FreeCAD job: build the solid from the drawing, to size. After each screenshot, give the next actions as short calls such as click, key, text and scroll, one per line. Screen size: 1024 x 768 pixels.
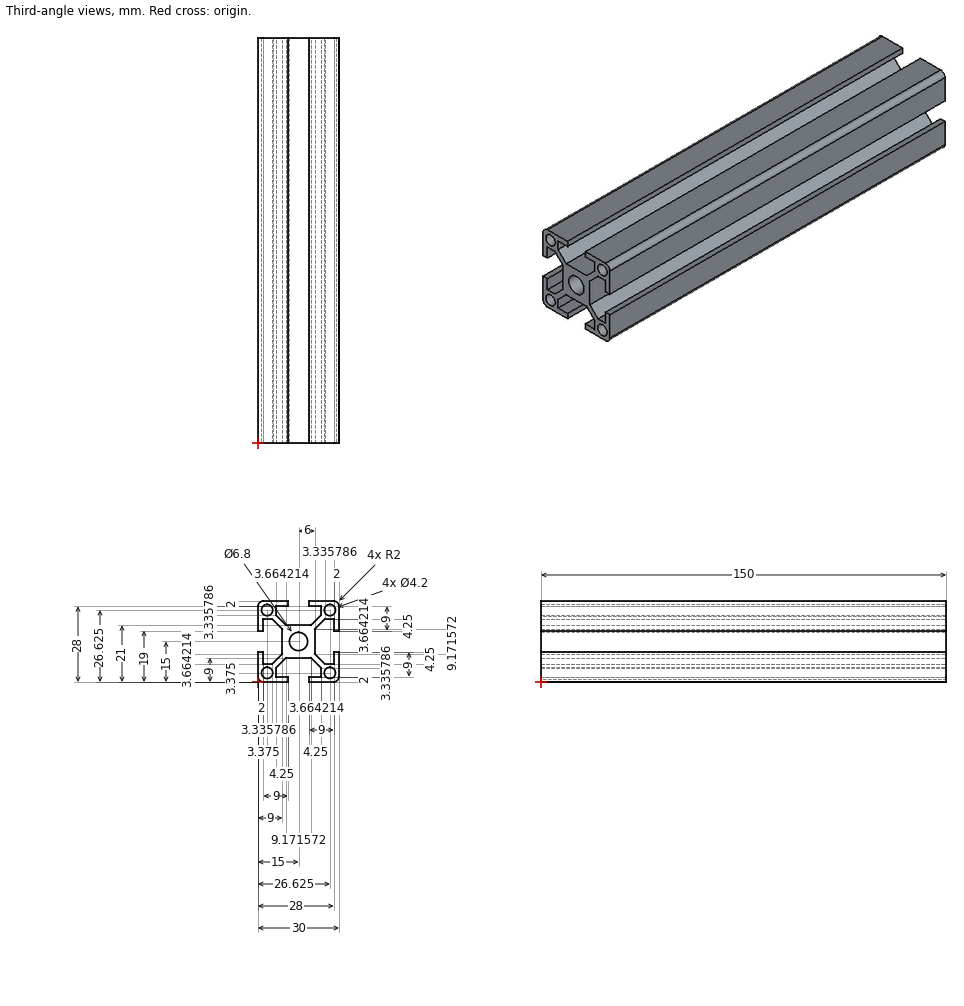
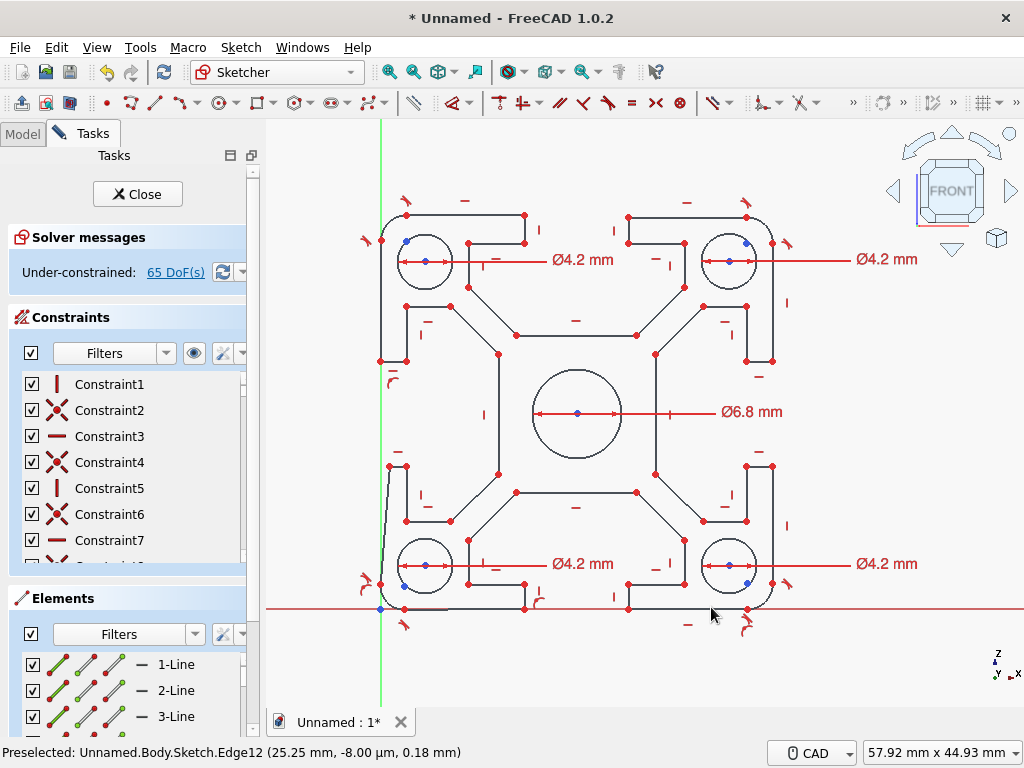
click(489, 609)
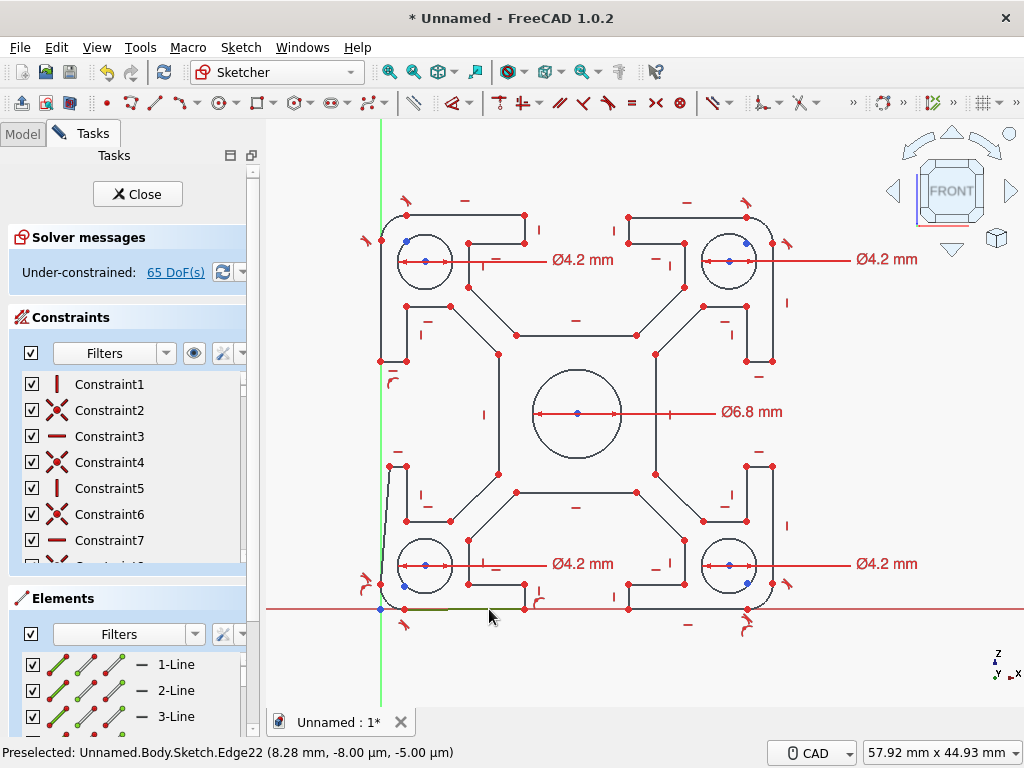
click(542, 104)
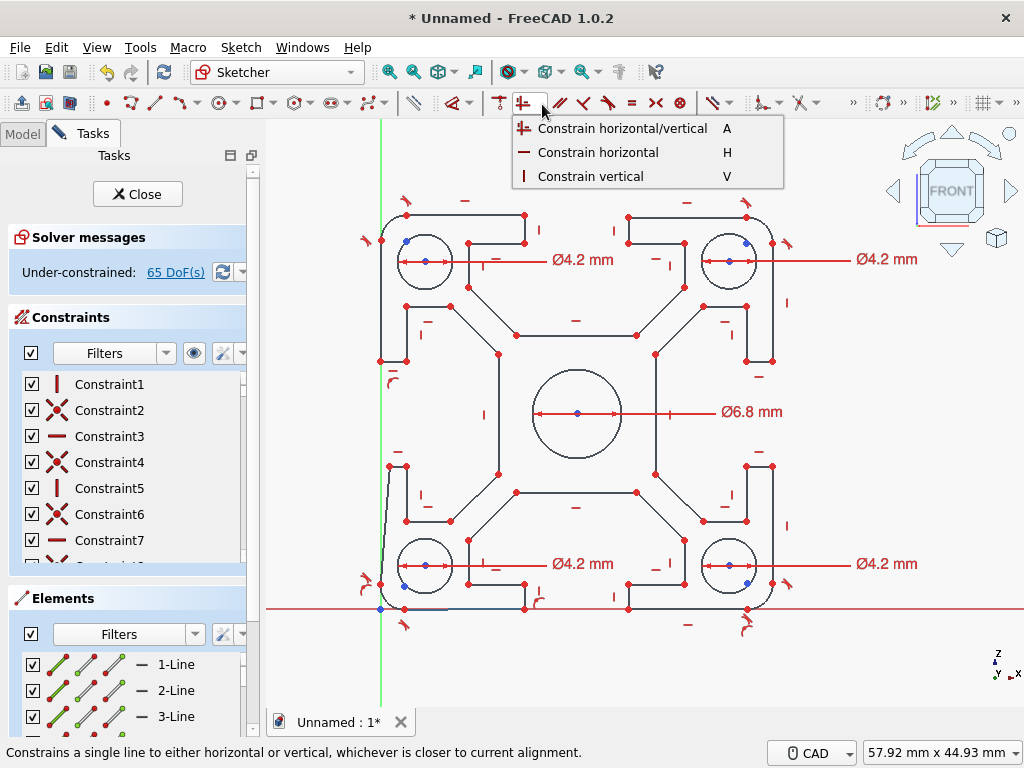
click(648, 152)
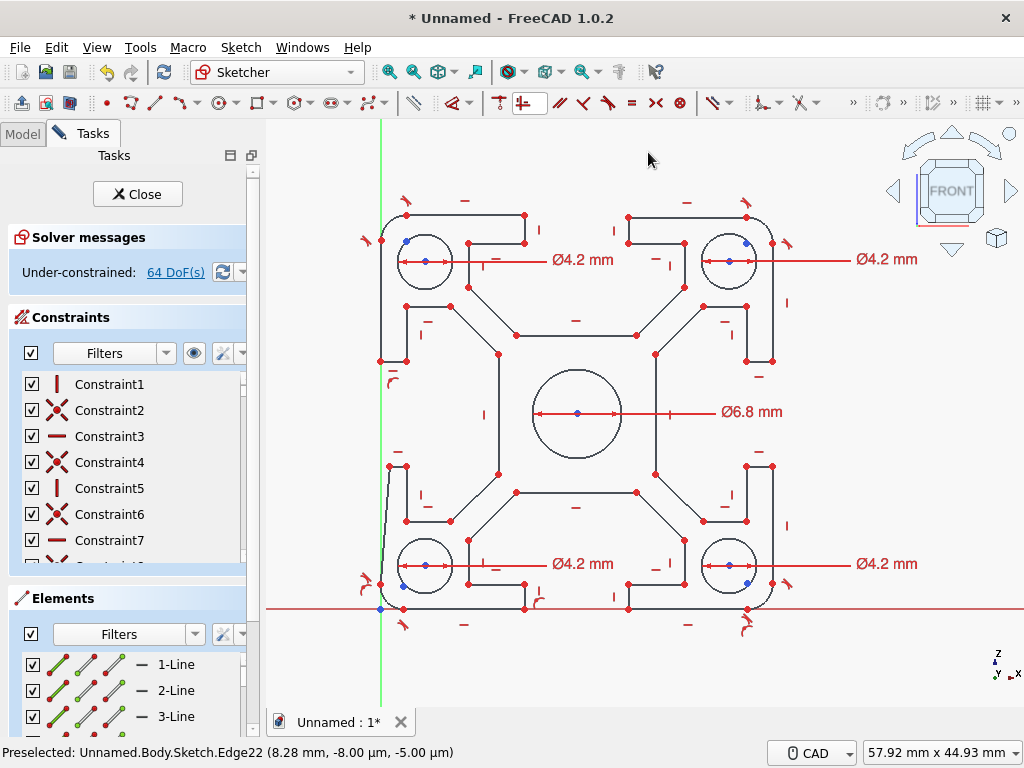
click(383, 549)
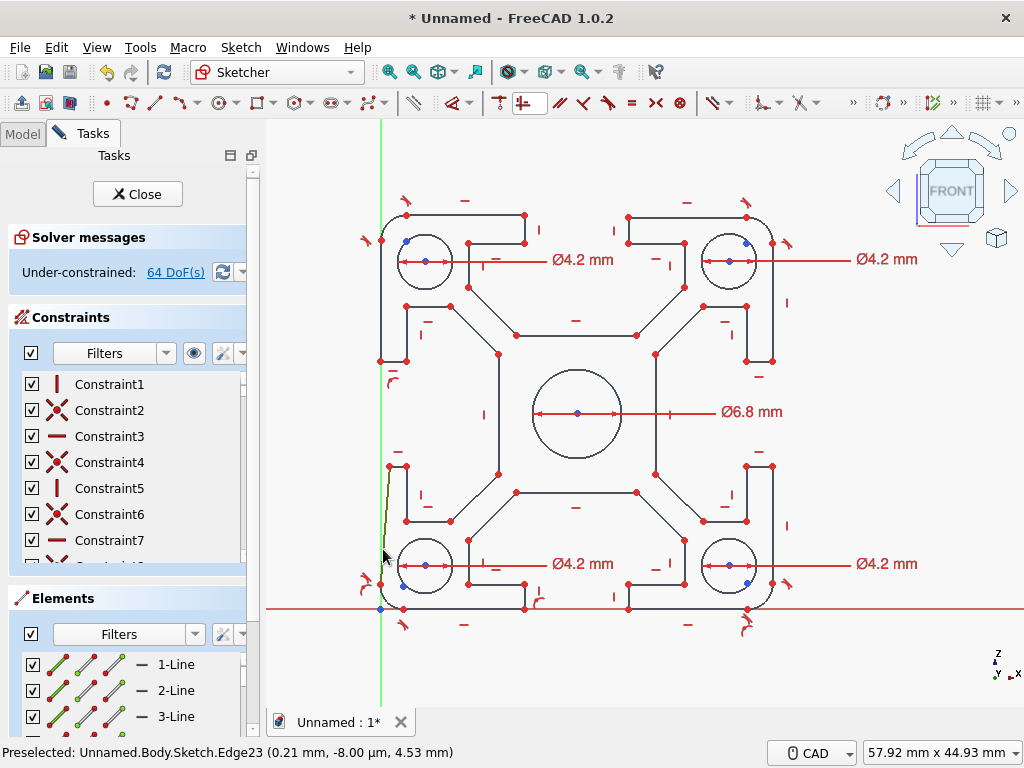
key(v)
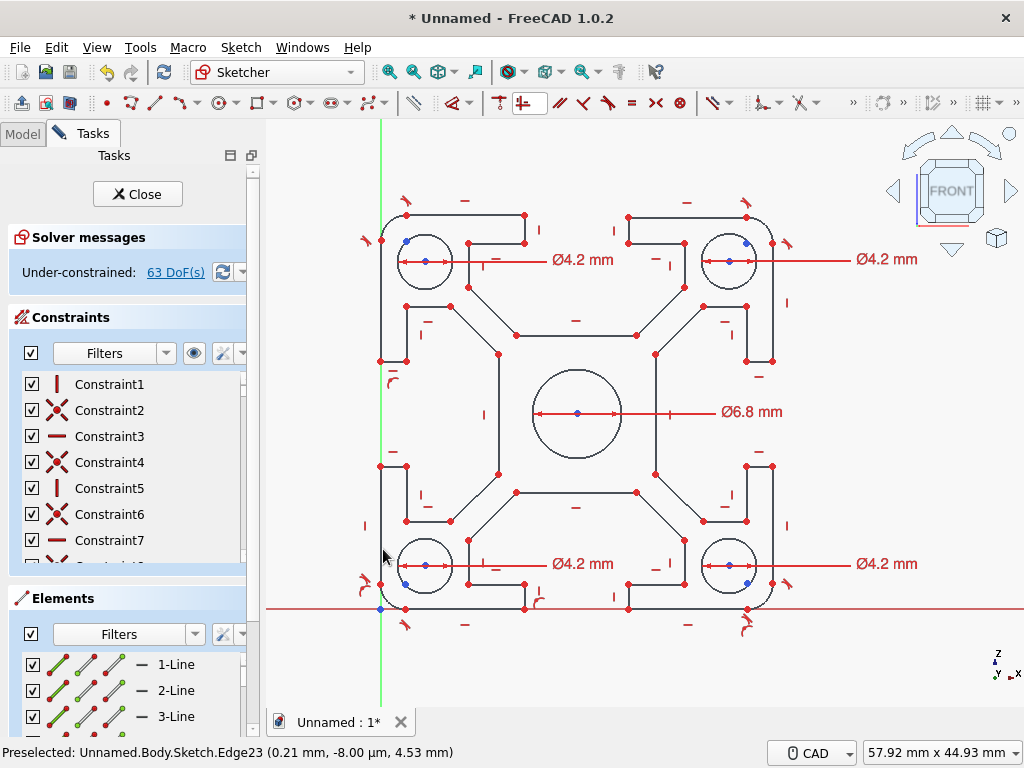
click(381, 325)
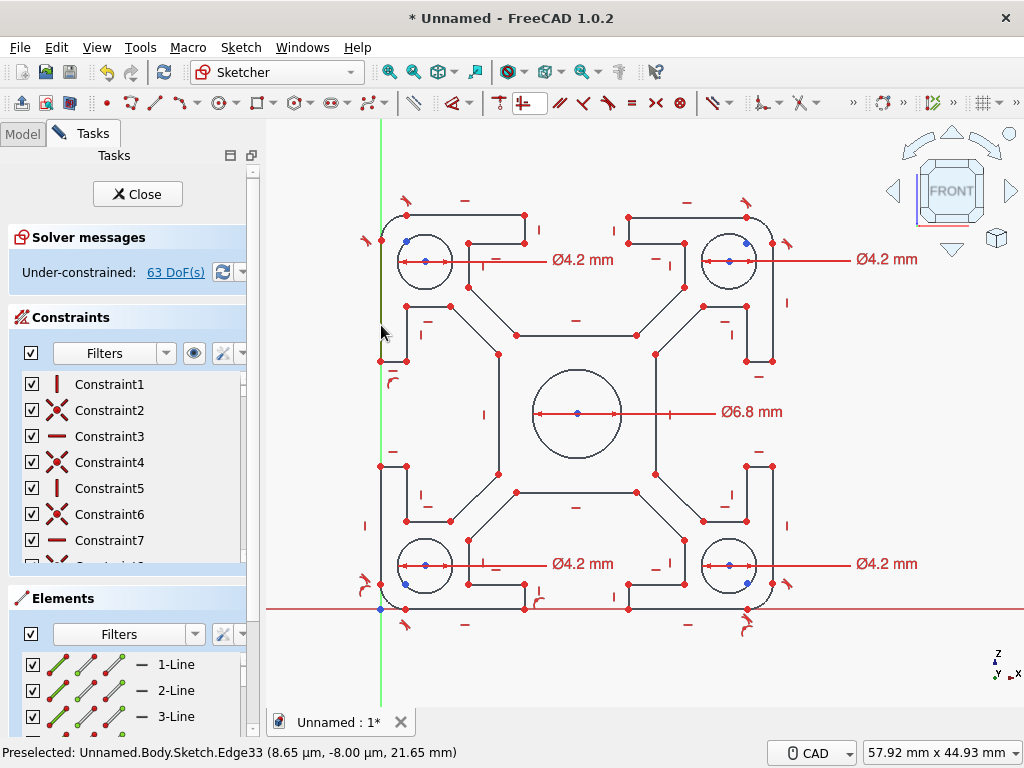
click(542, 104)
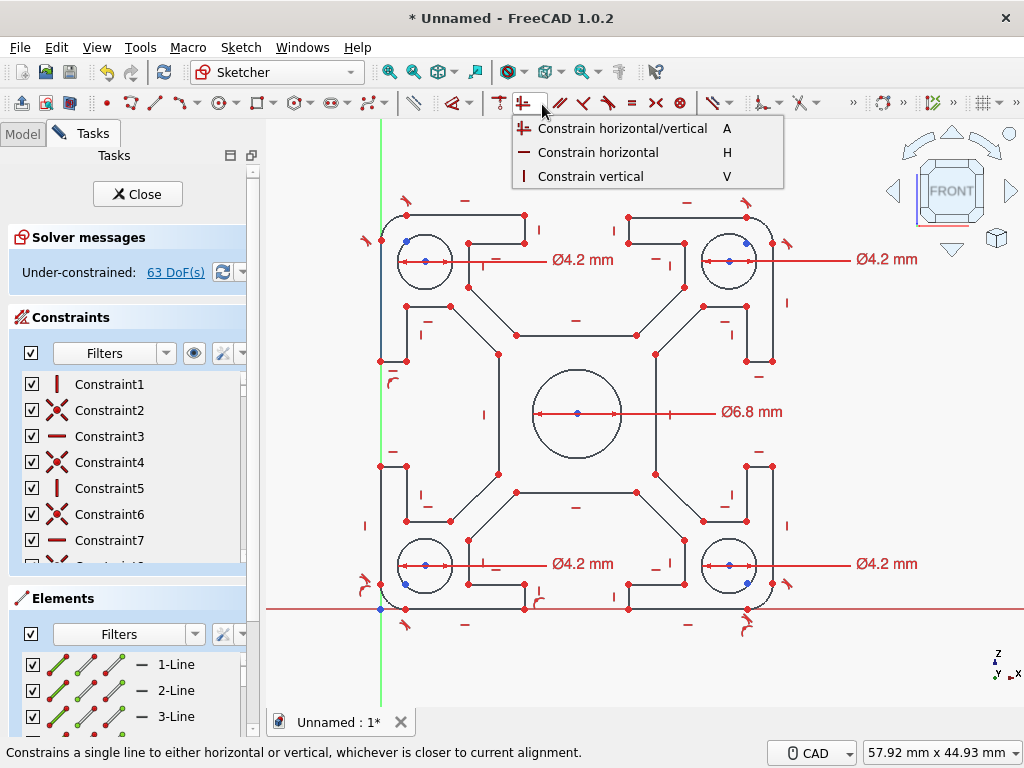
click(648, 176)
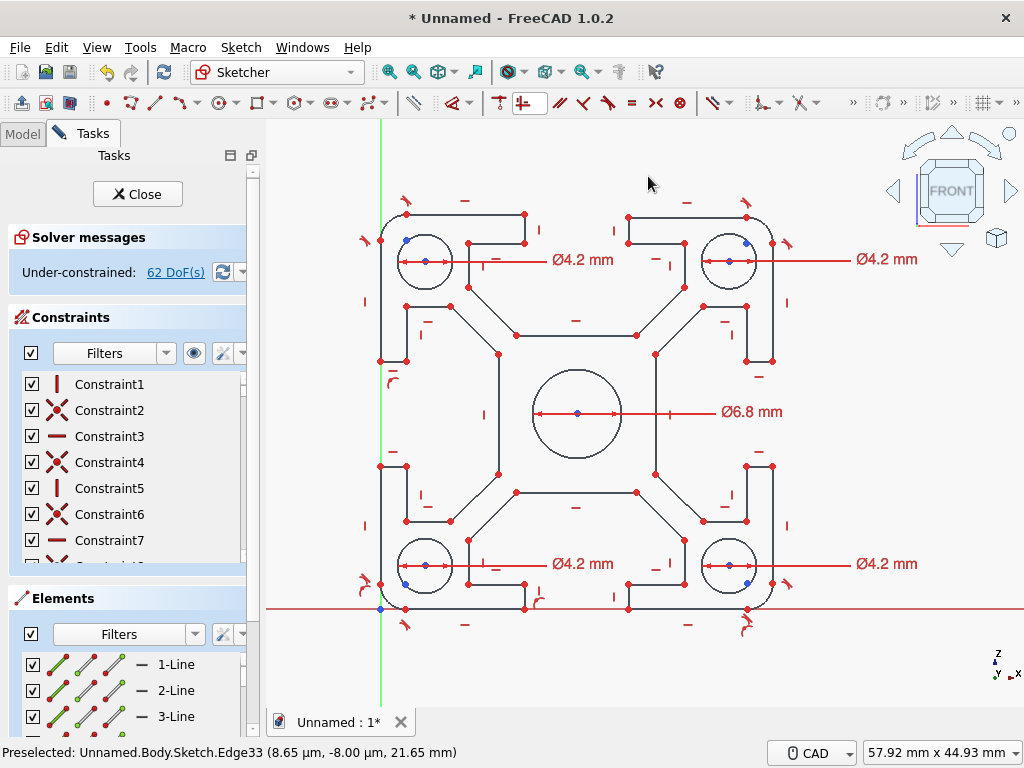
click(759, 607)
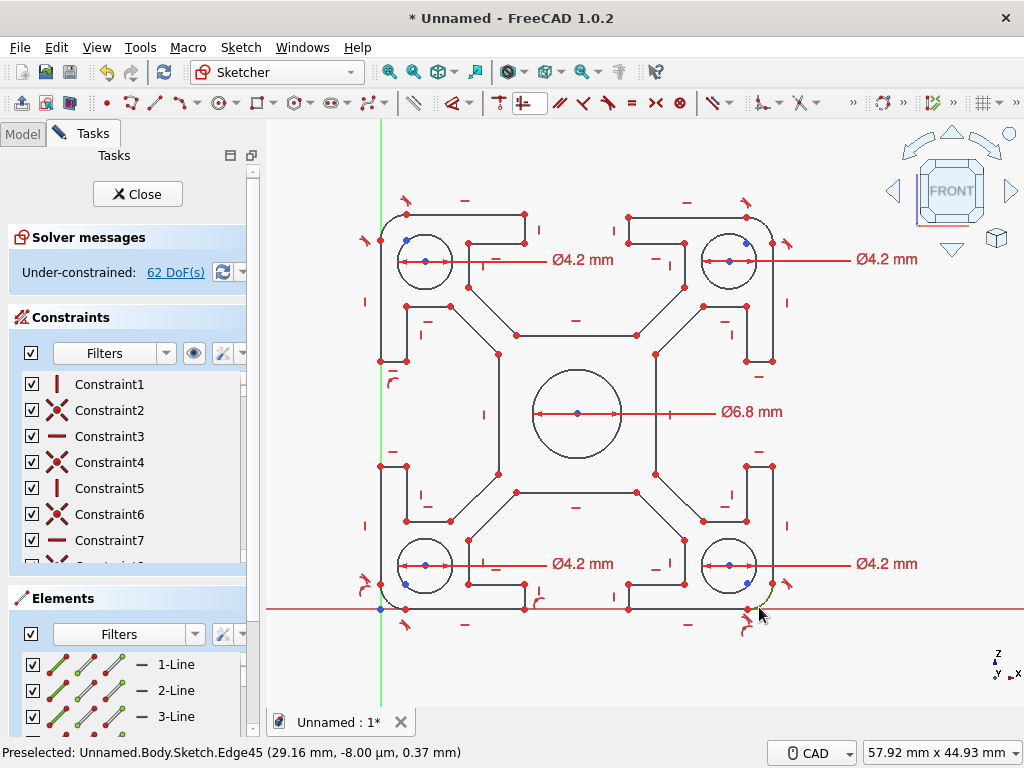
click(383, 596)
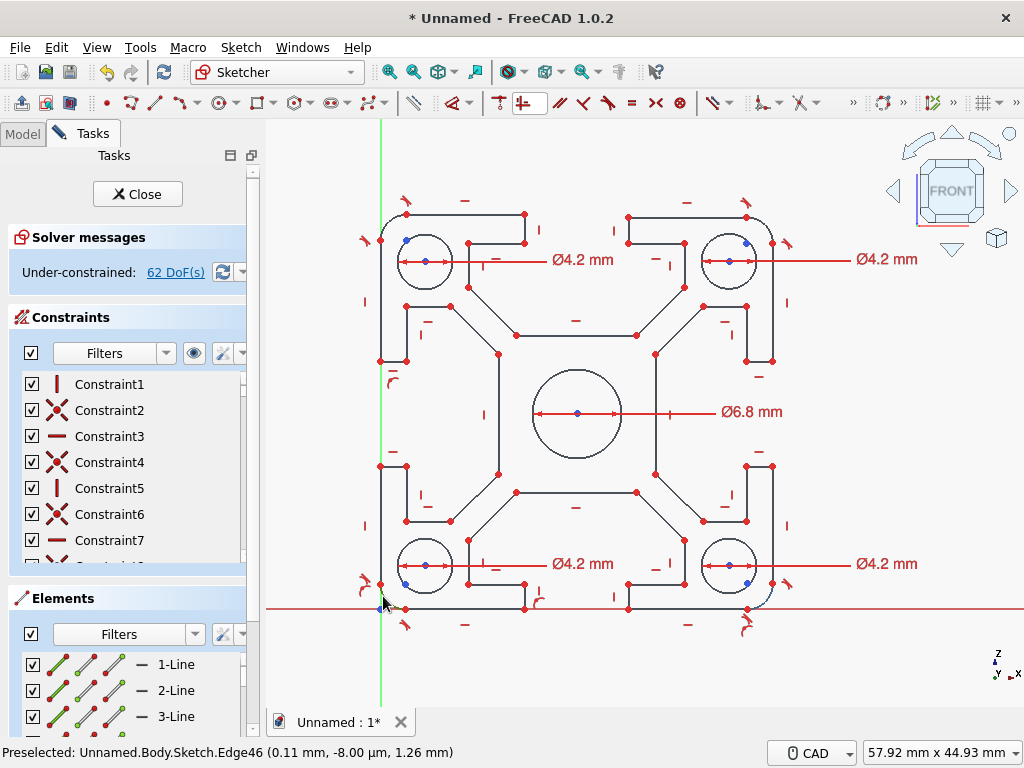
click(395, 218)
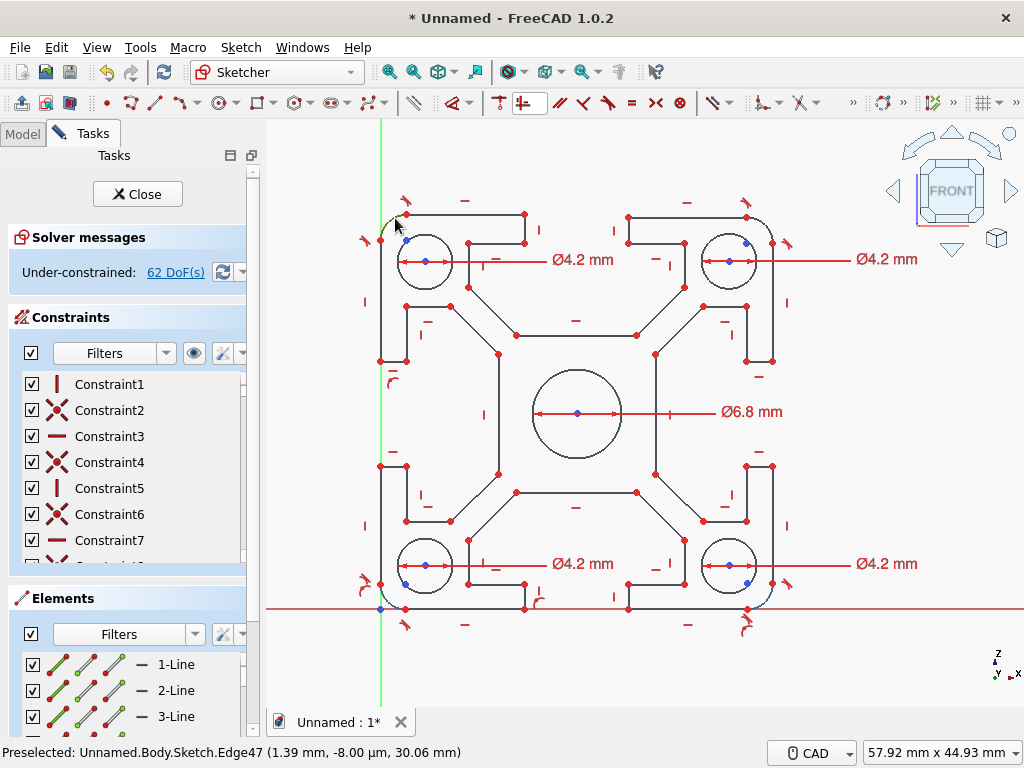
click(770, 232)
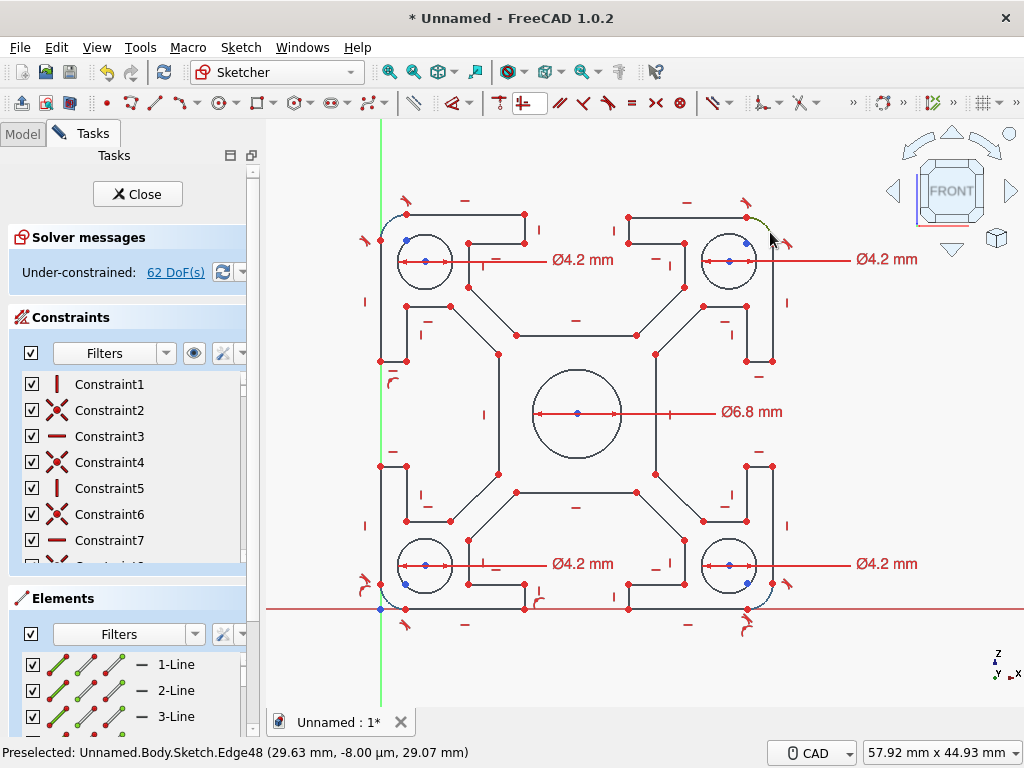
key(e)